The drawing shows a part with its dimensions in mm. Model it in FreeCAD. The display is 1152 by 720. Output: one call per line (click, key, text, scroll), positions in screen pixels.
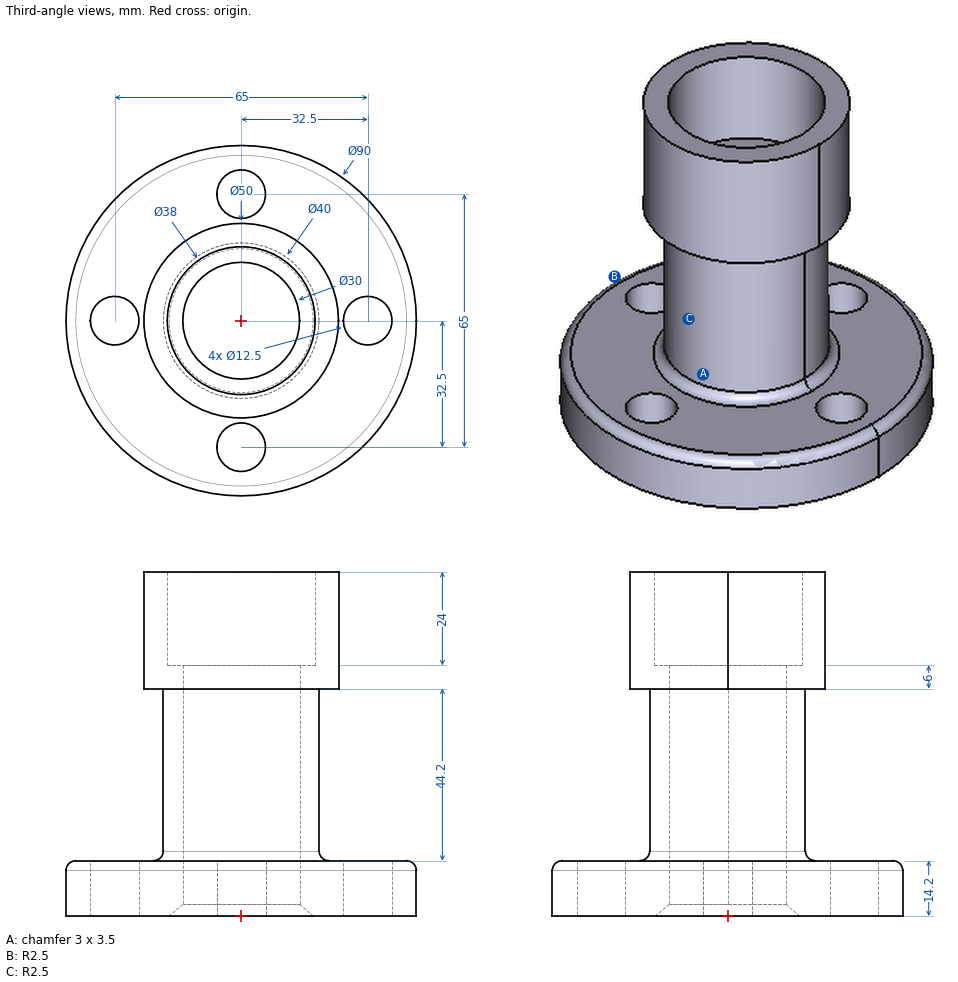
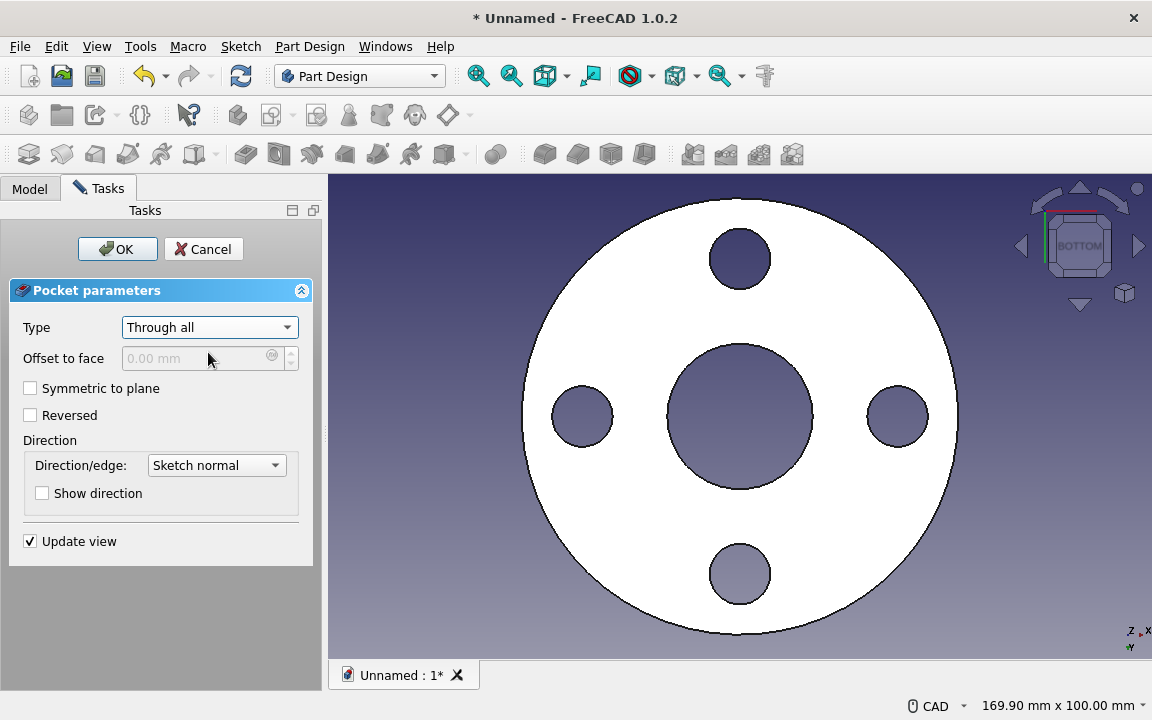
click(118, 249)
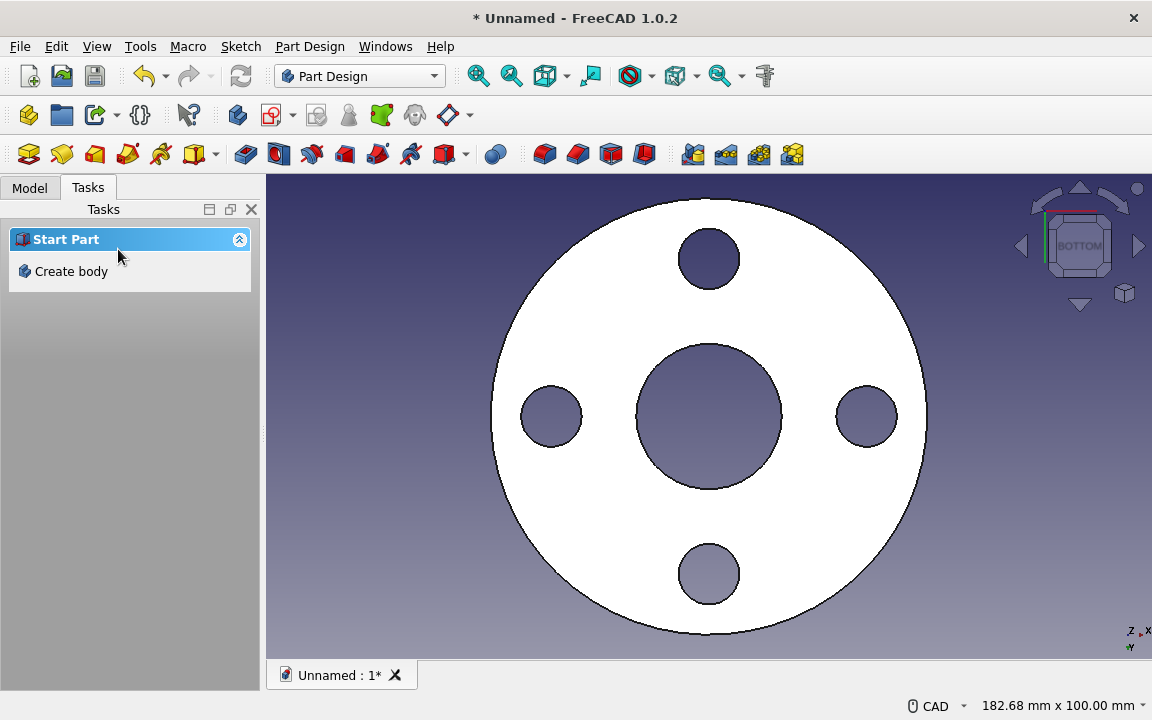
click(650, 373)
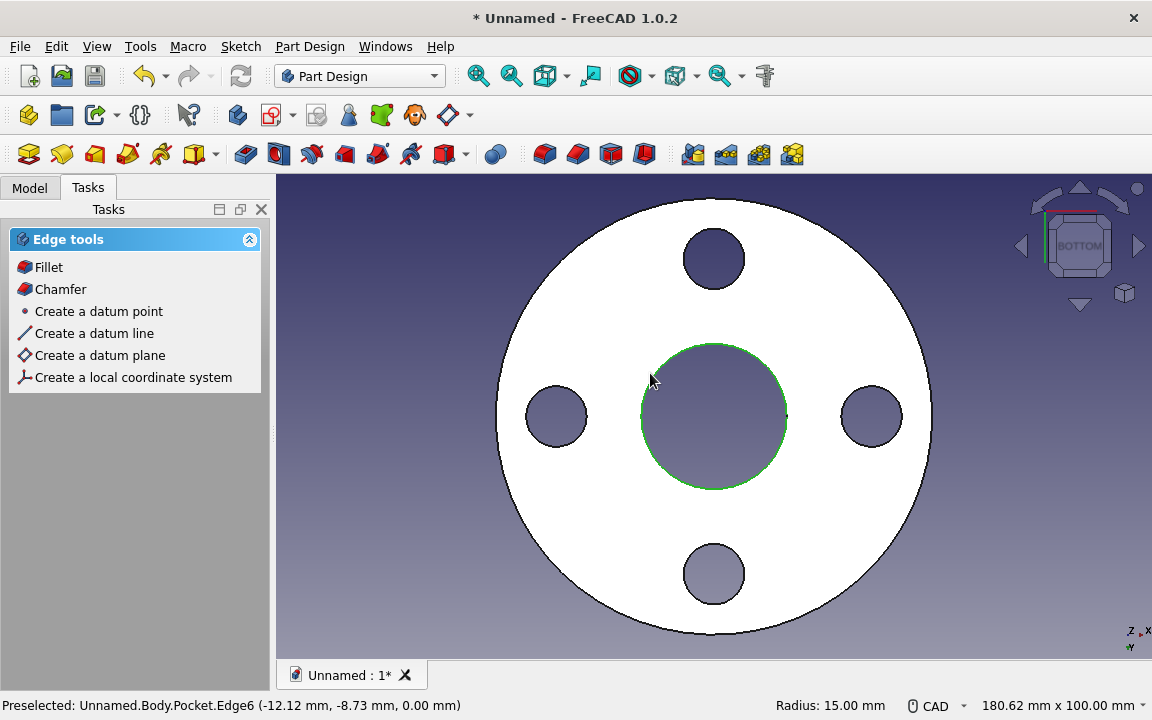
click(578, 154)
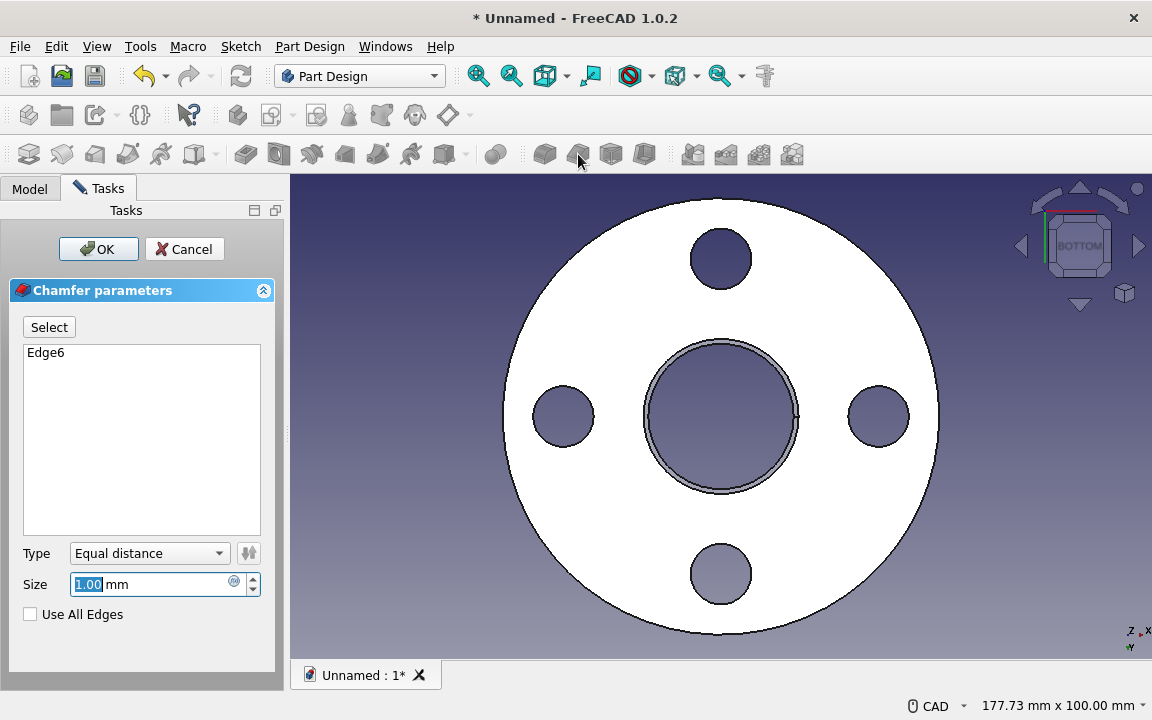
text(3)
key(Tab)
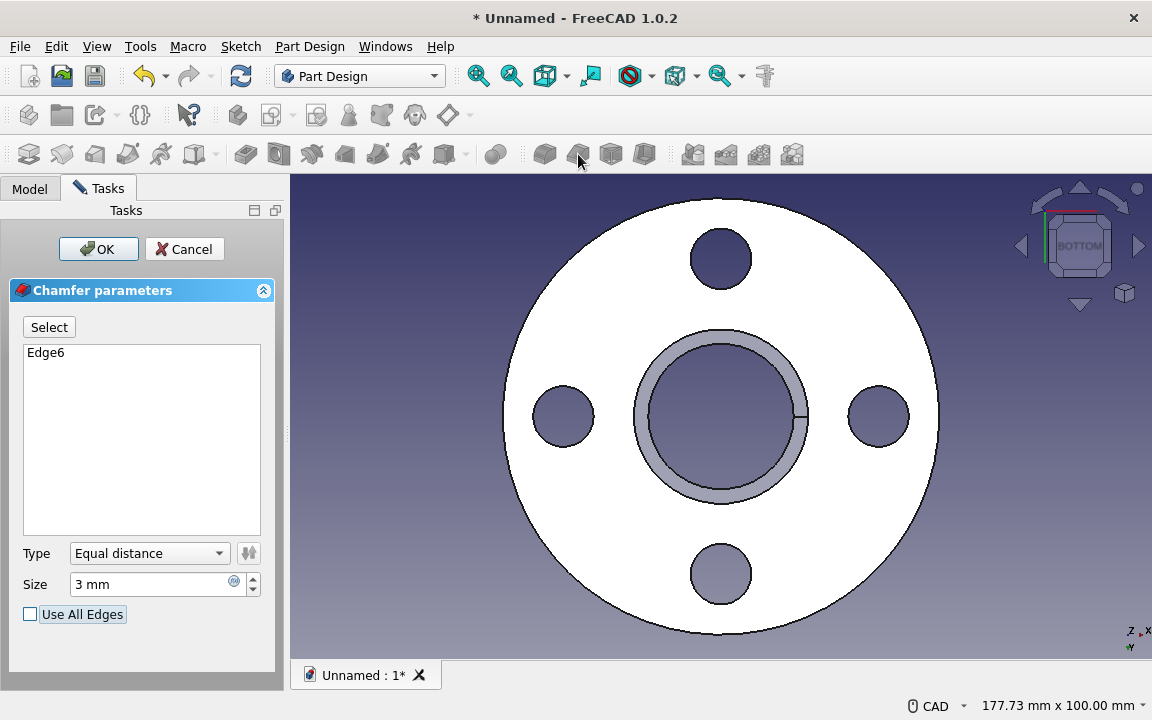
click(150, 554)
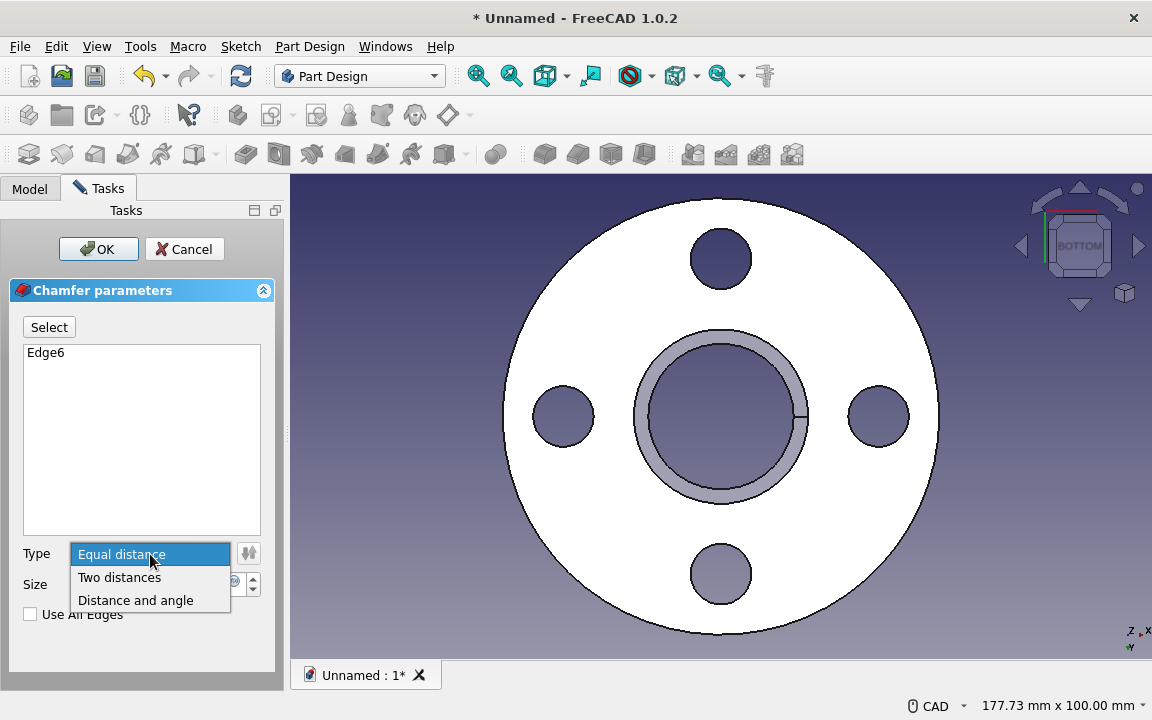
click(148, 578)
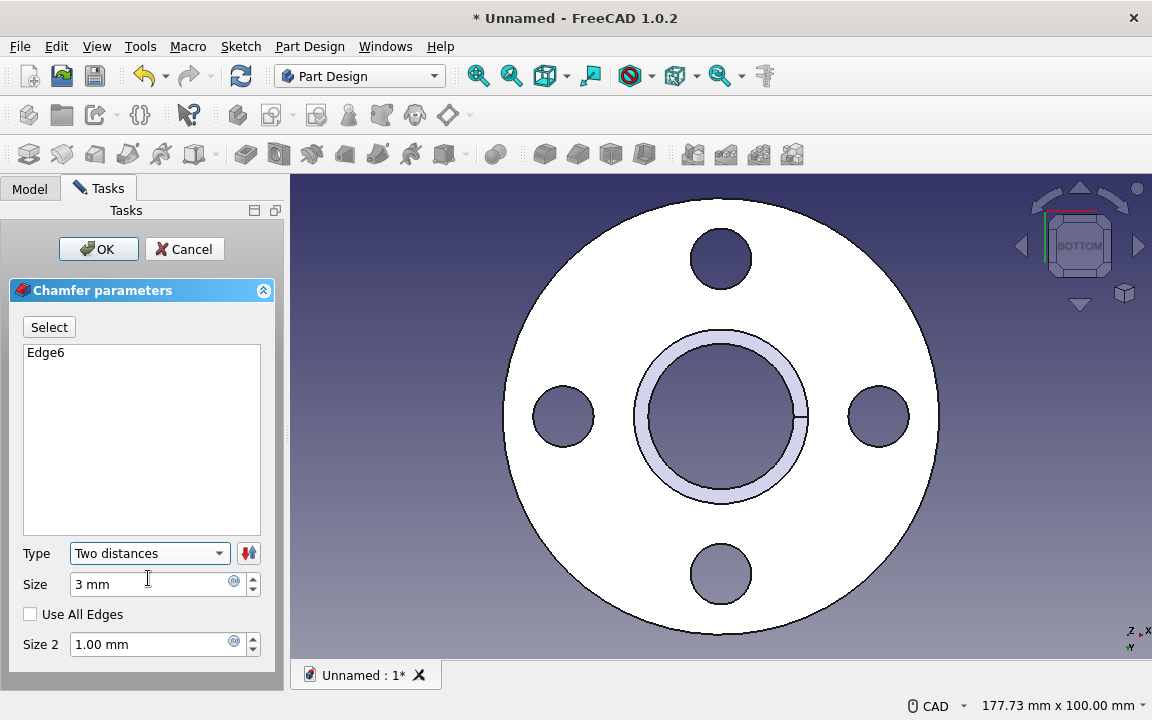
triple_click(158, 644)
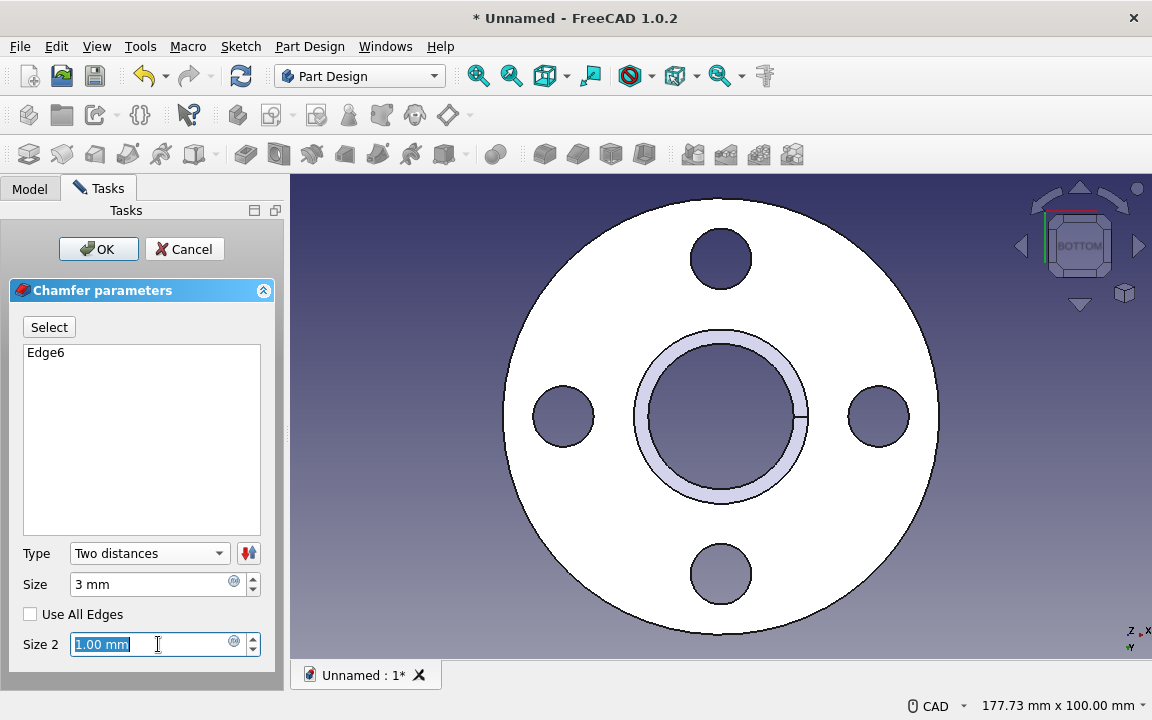
text(3.5)
key(Tab)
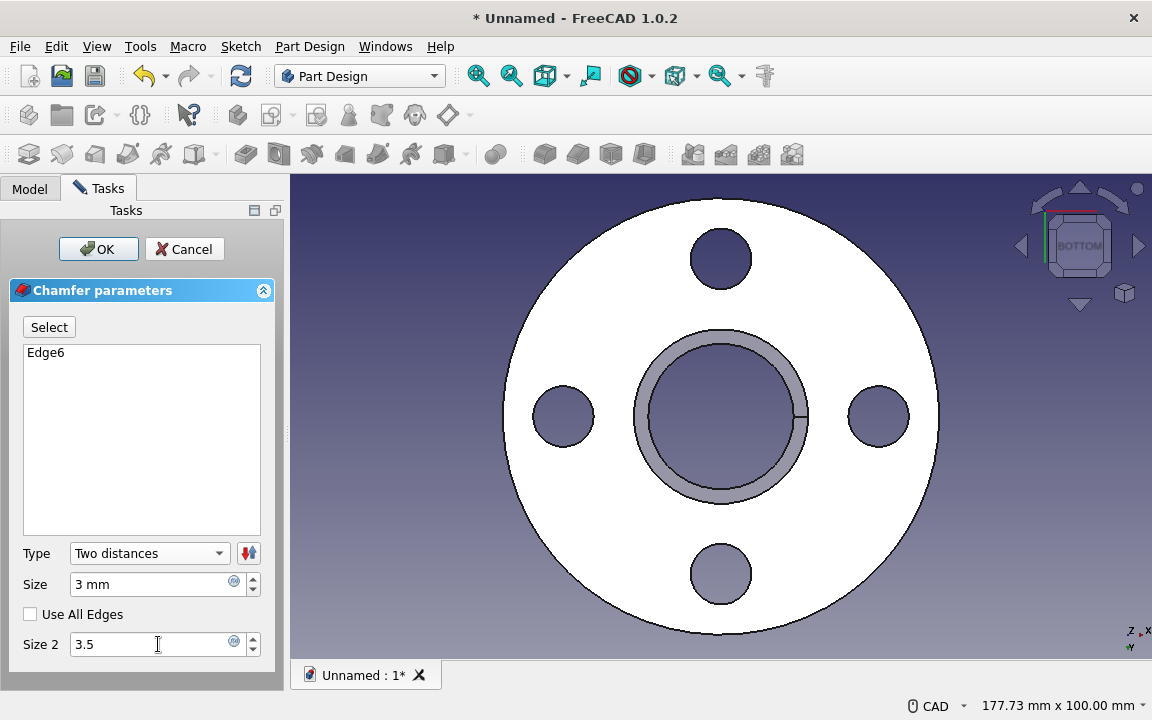
click(249, 554)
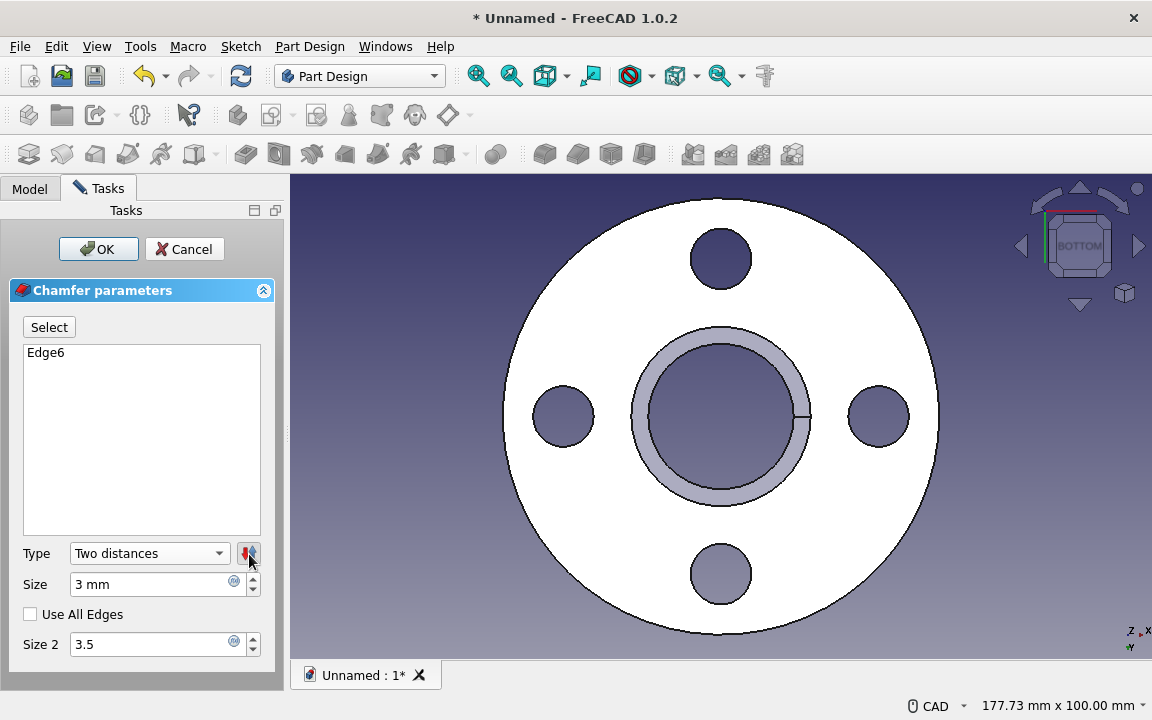
click(99, 249)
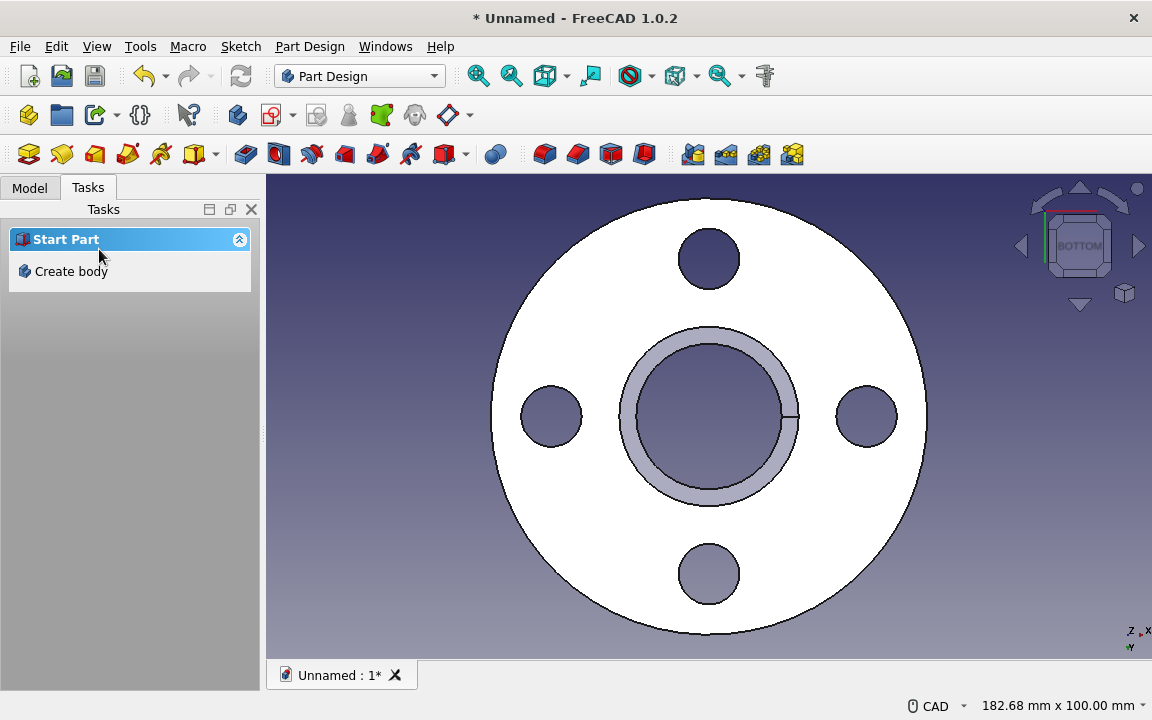
key(0)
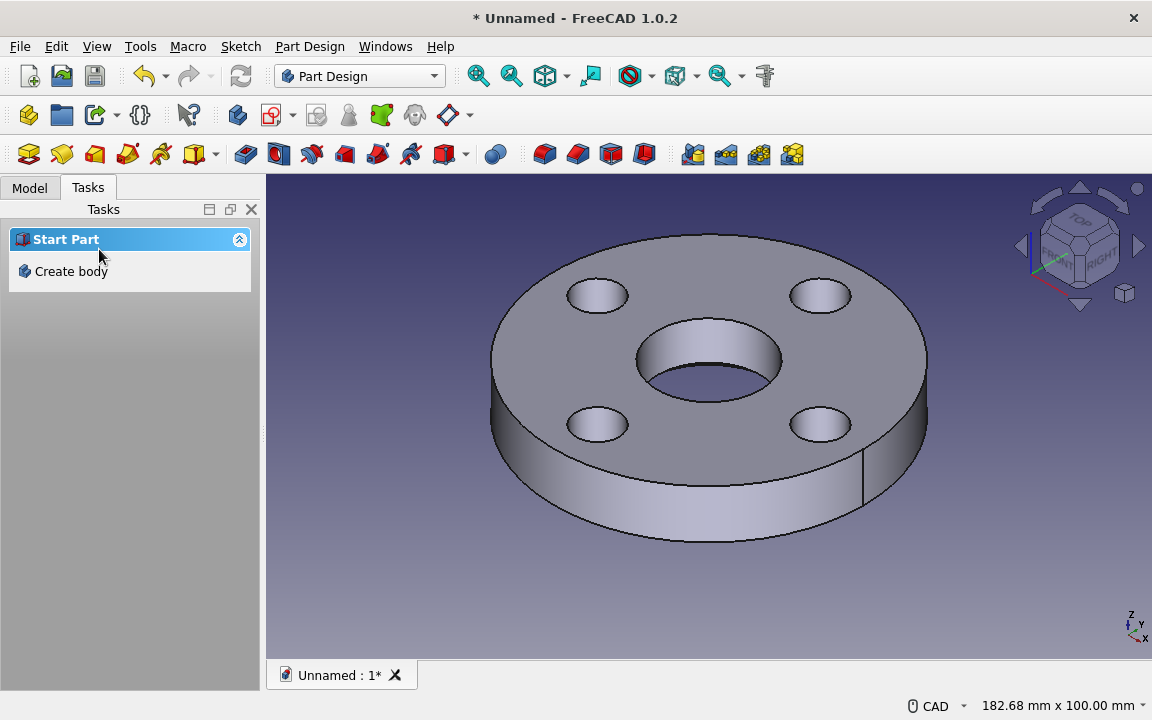
click(885, 359)